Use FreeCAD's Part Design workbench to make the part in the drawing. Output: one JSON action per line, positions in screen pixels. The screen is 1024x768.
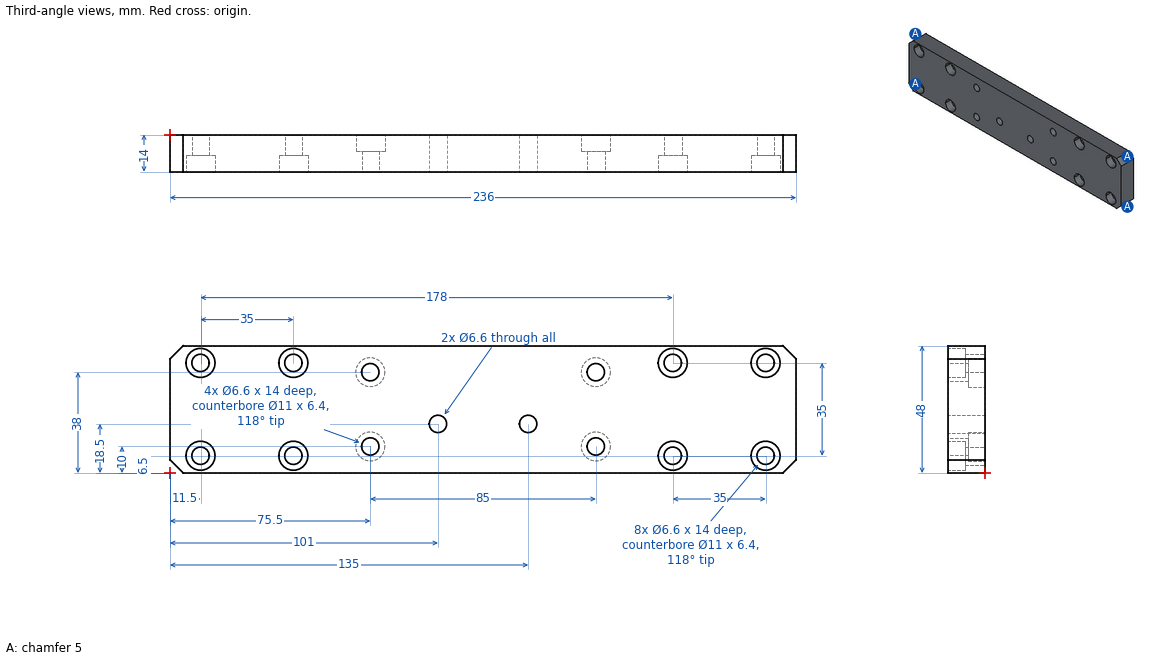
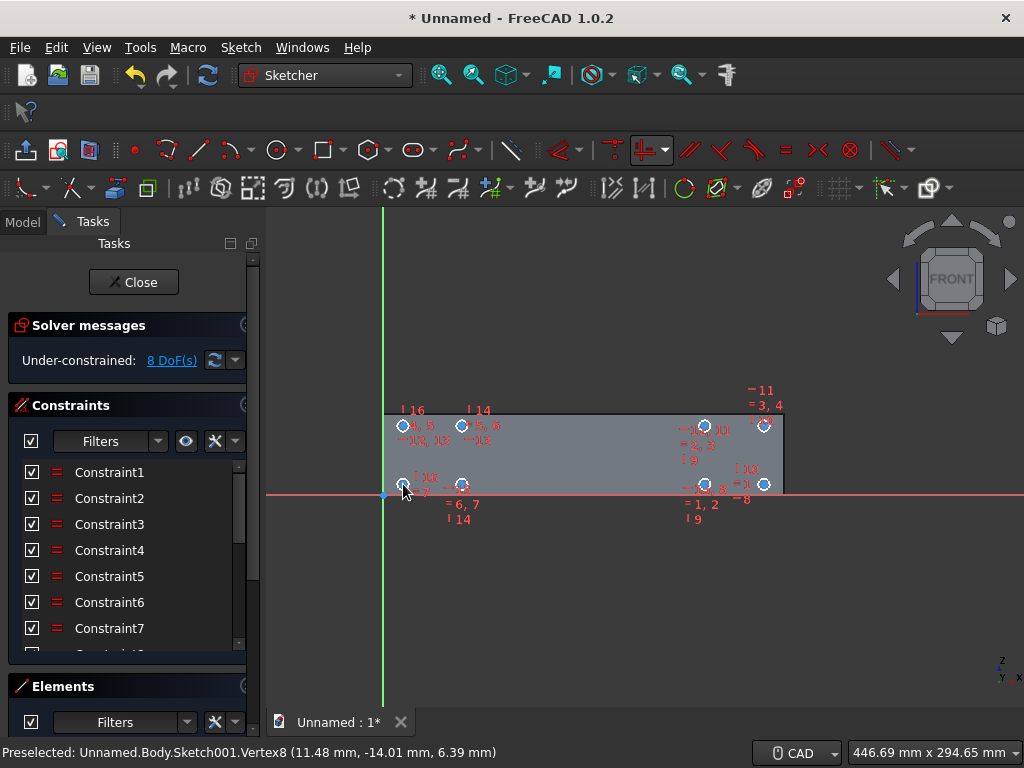
{"action": "scroll", "coordinate": [462, 484], "scroll_direction": "up", "scroll_amount": 4}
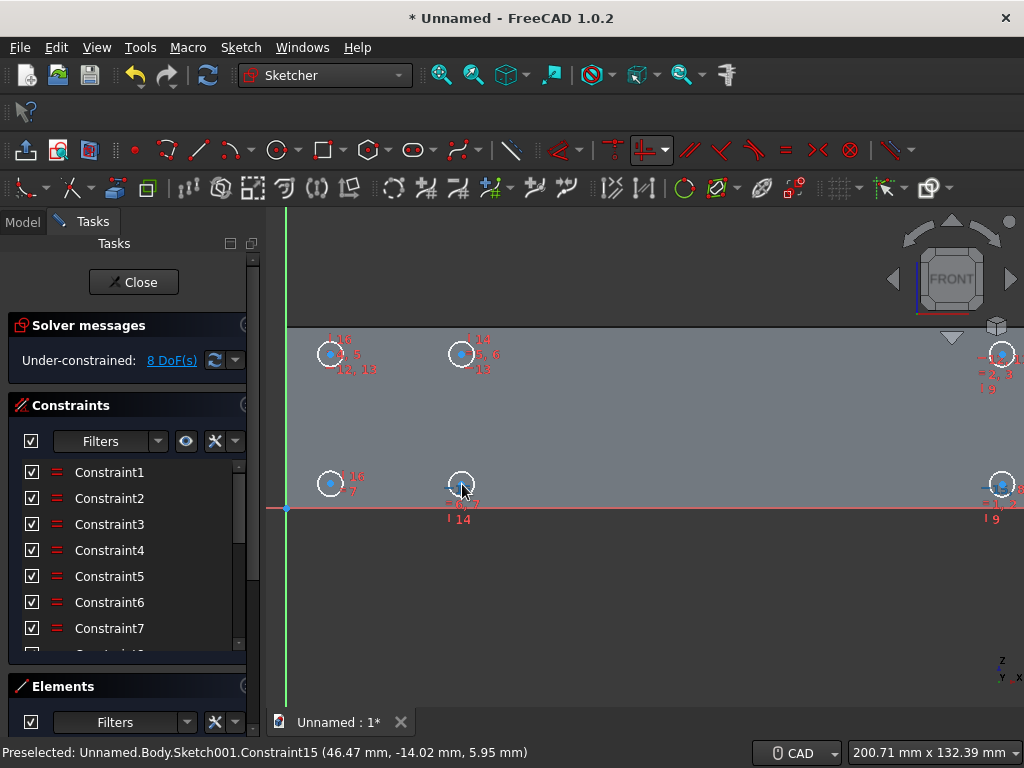
{"action": "scroll", "coordinate": [462, 484], "scroll_direction": "up", "scroll_amount": 4}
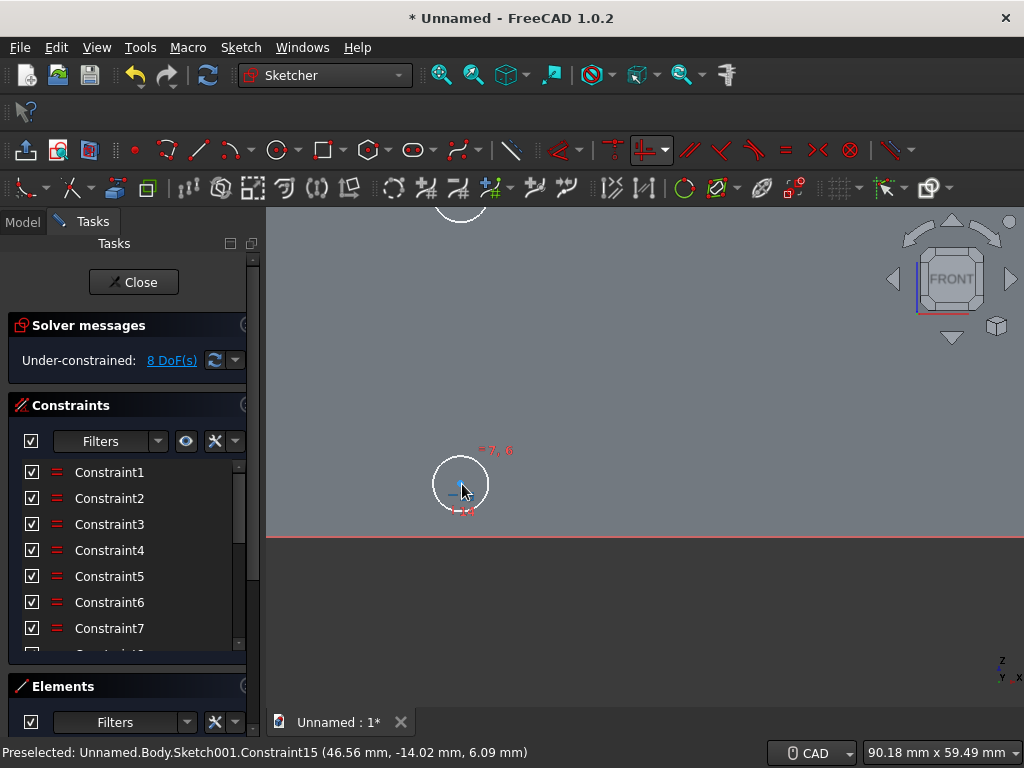
{"action": "left_click", "coordinate": [461, 484]}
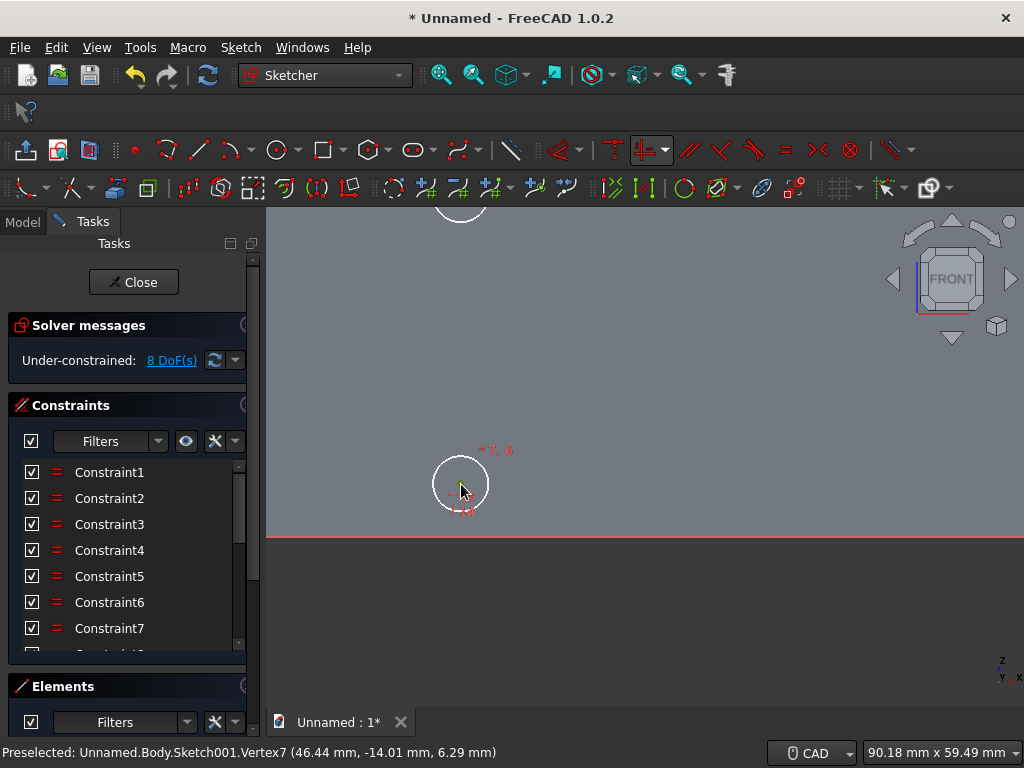
{"action": "scroll", "coordinate": [462, 484], "scroll_direction": "down", "scroll_amount": 8}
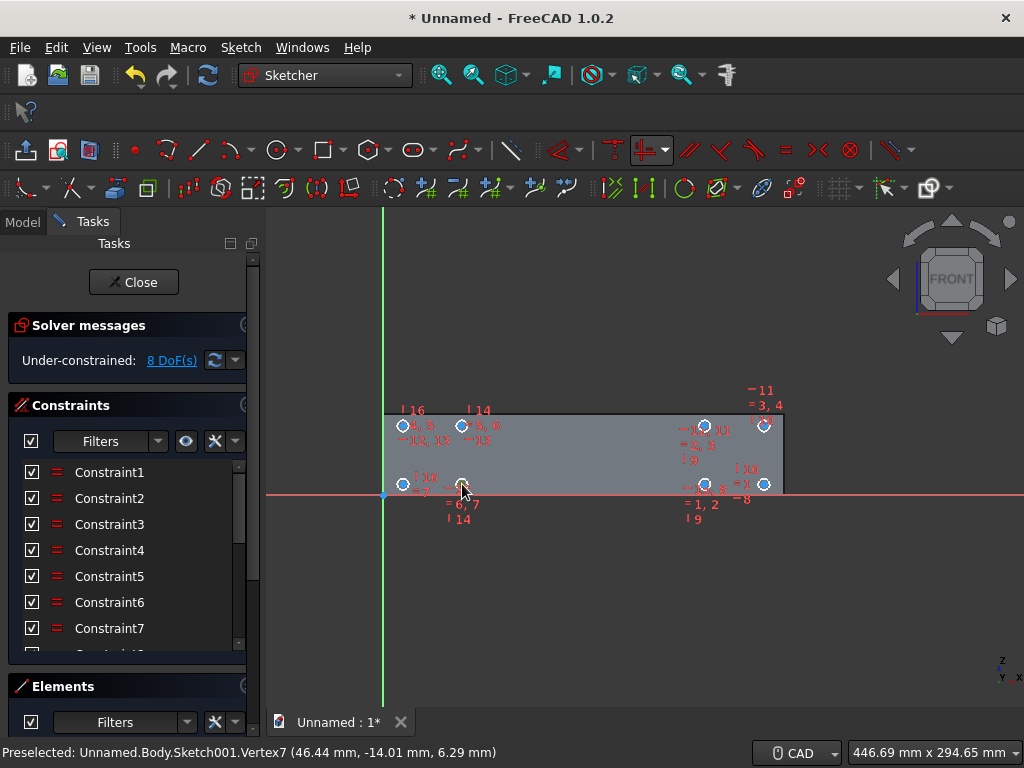
{"action": "left_click", "coordinate": [403, 484]}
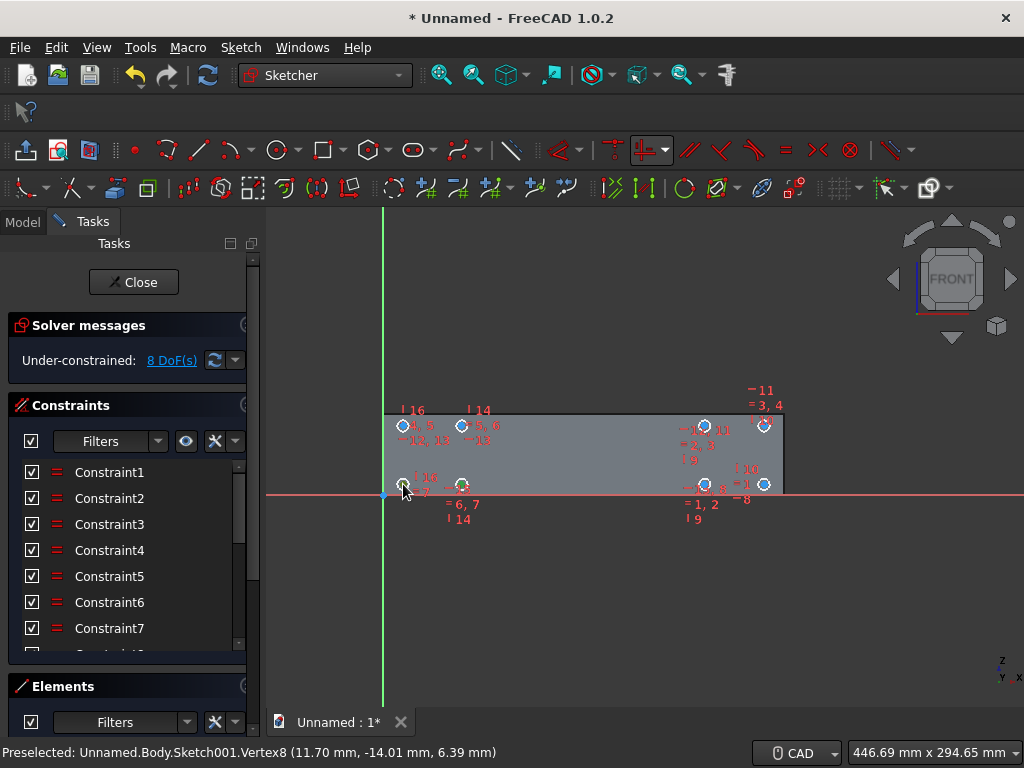
{"action": "left_click", "coordinate": [668, 150]}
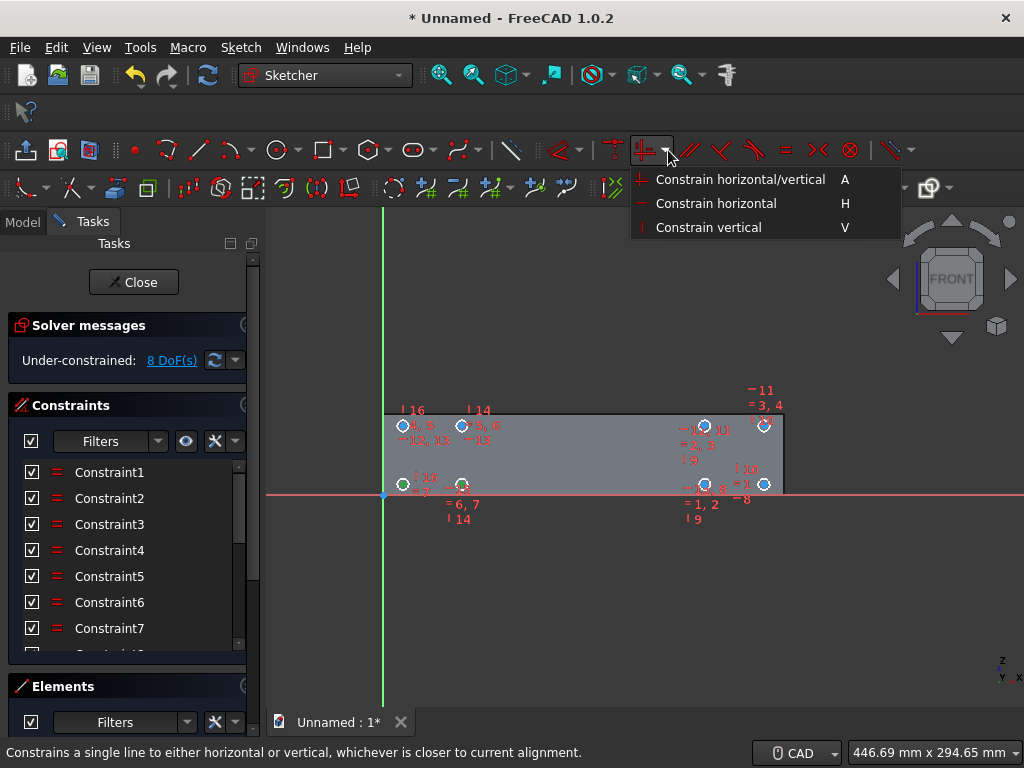
{"action": "left_click", "coordinate": [766, 203]}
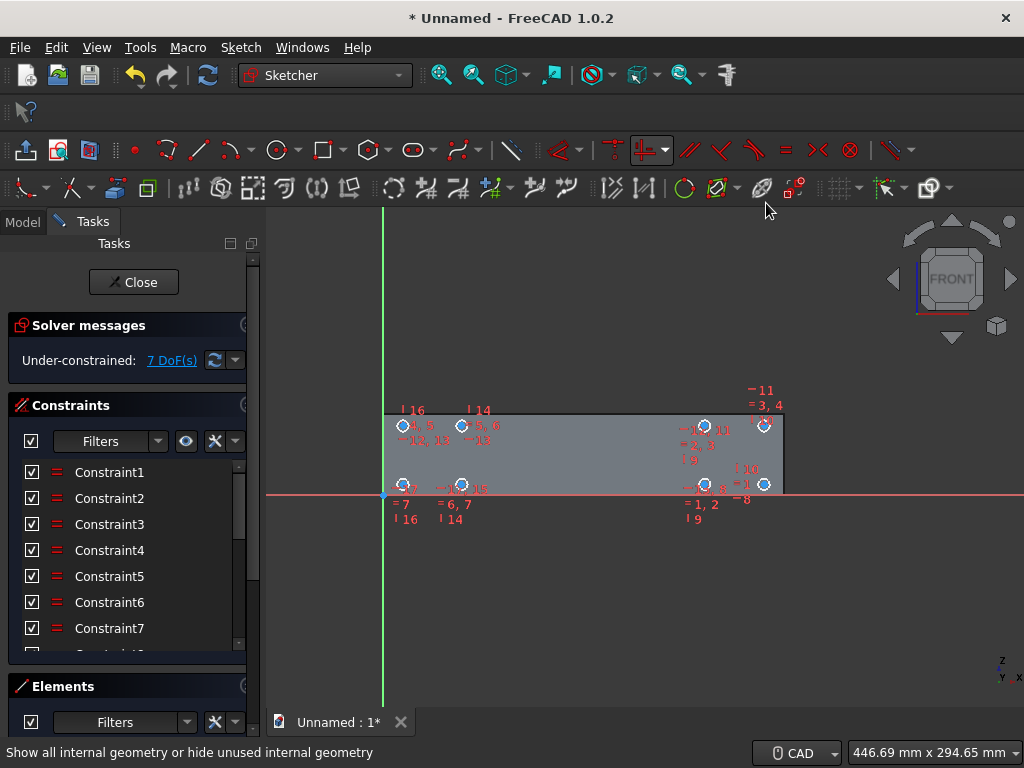
{"action": "left_click", "coordinate": [558, 150]}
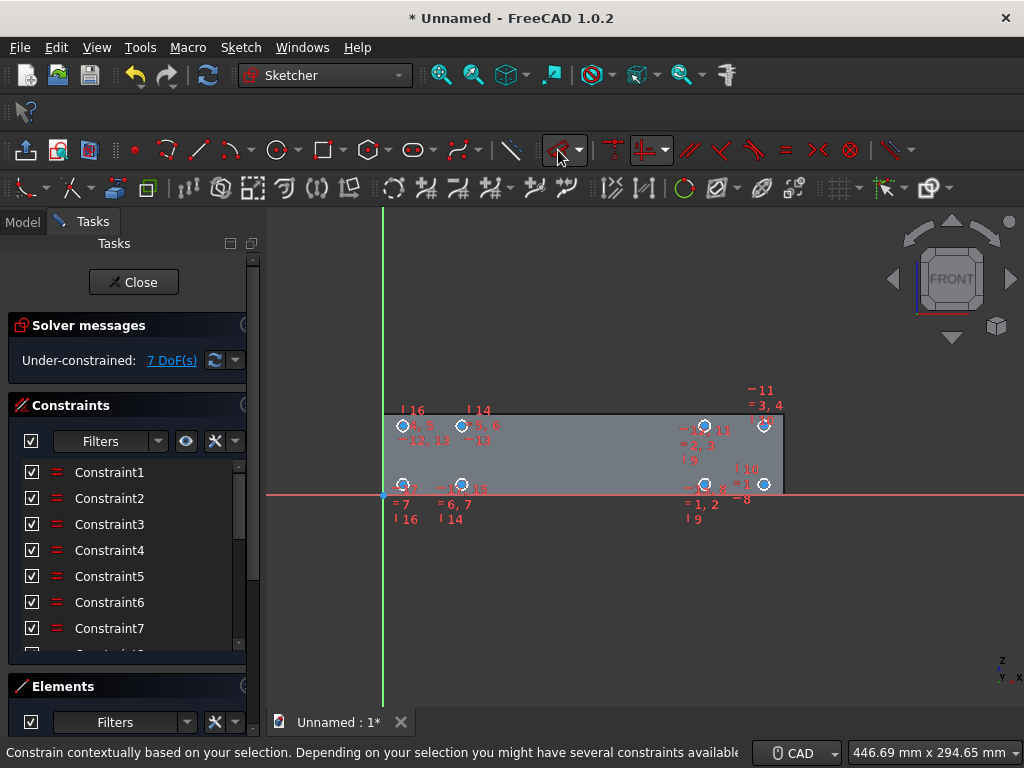
{"action": "scroll", "coordinate": [768, 488], "scroll_direction": "up", "scroll_amount": 7}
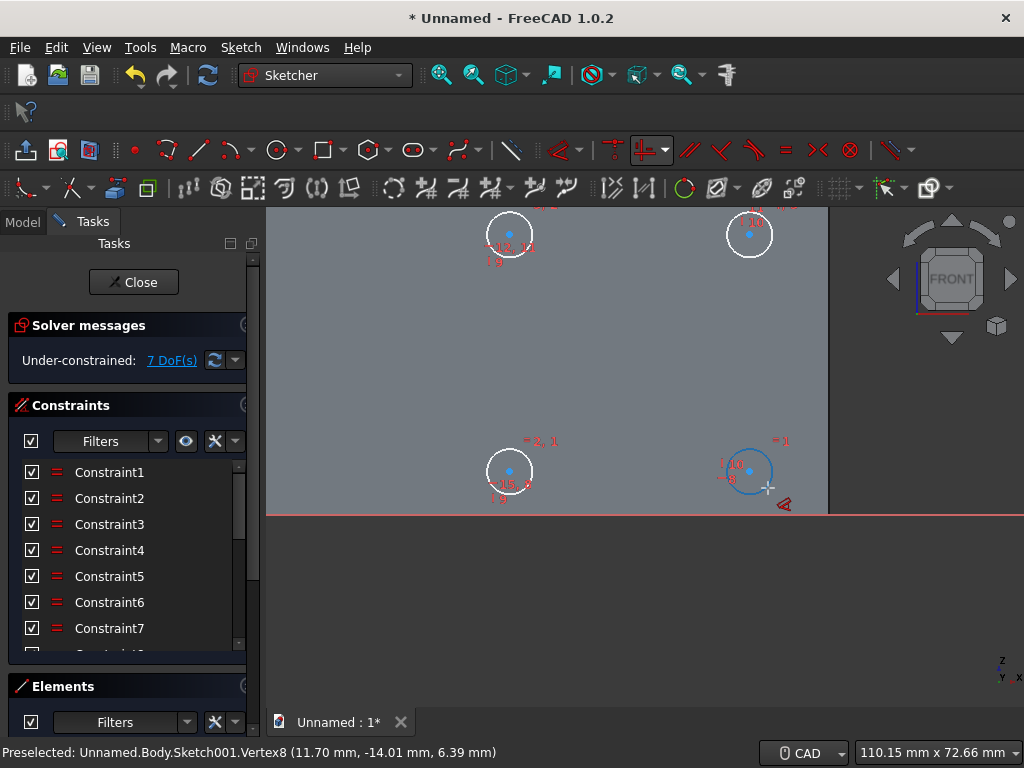
{"action": "left_click", "coordinate": [766, 488]}
{"action": "left_click", "coordinate": [803, 487]}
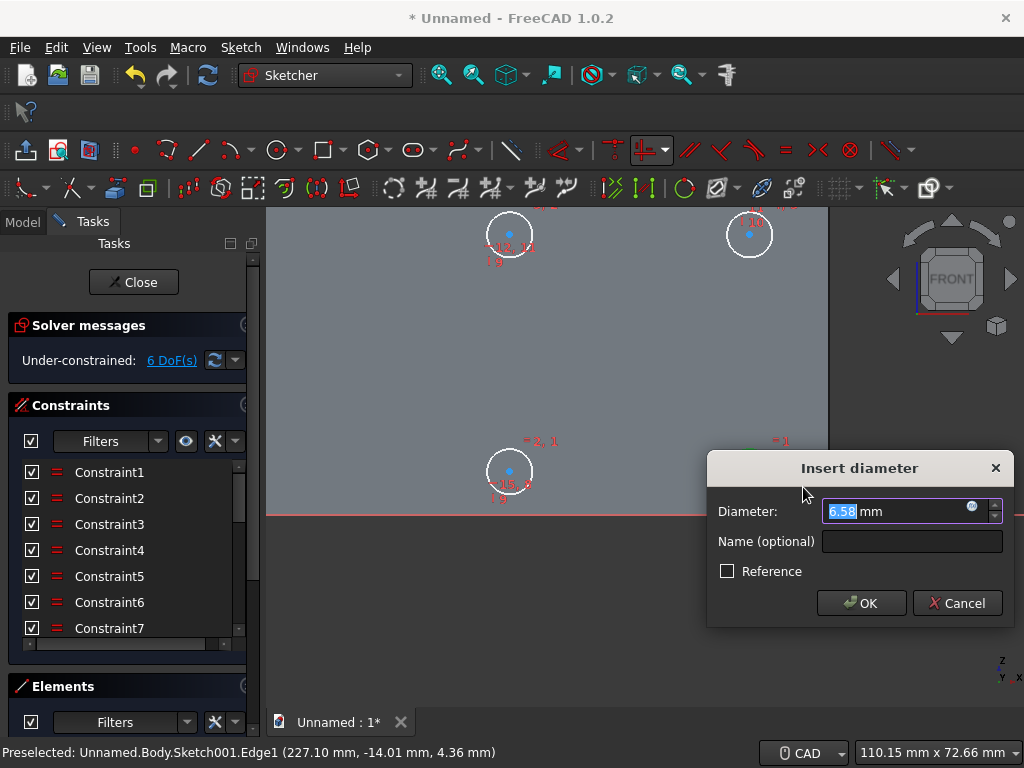
{"action": "type", "text": "6.6"}
{"action": "key", "text": "Return"}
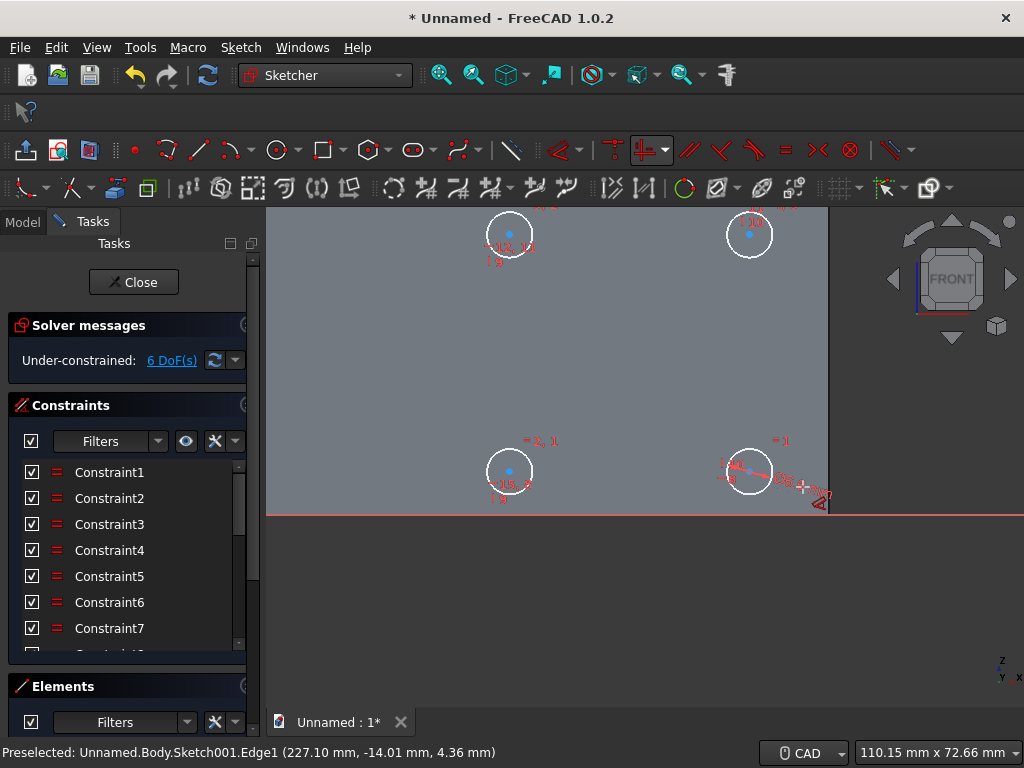
{"action": "left_click", "coordinate": [750, 472]}
{"action": "left_click", "coordinate": [784, 503]}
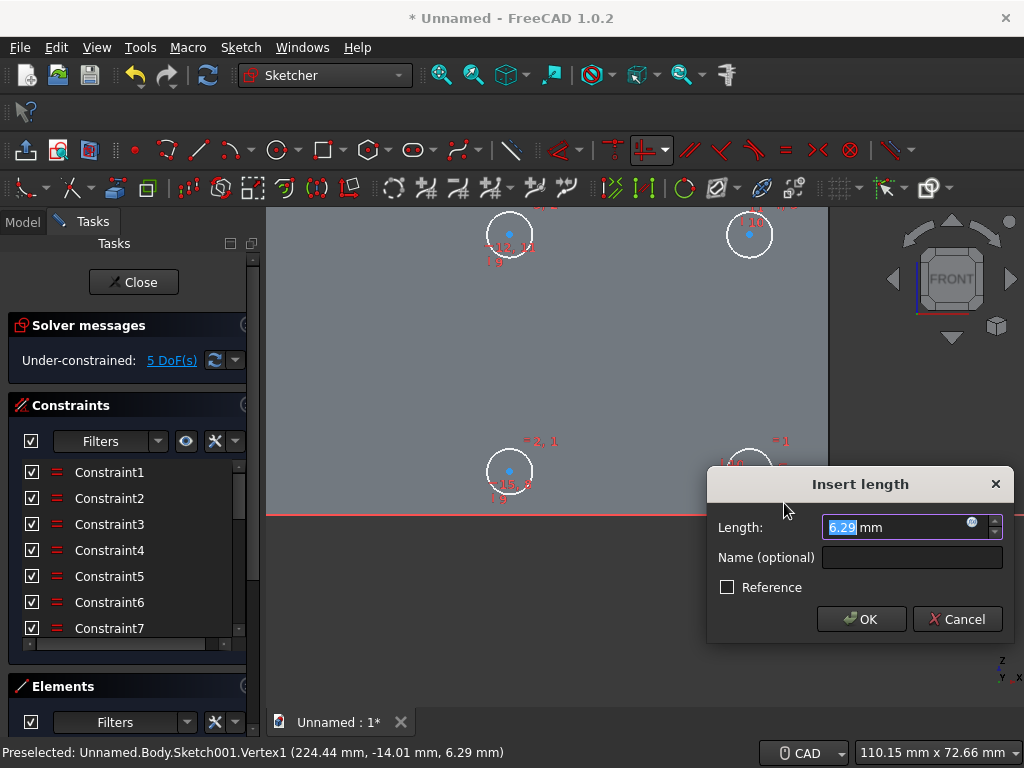
{"action": "type", "text": "6.5"}
{"action": "key", "text": "Return"}